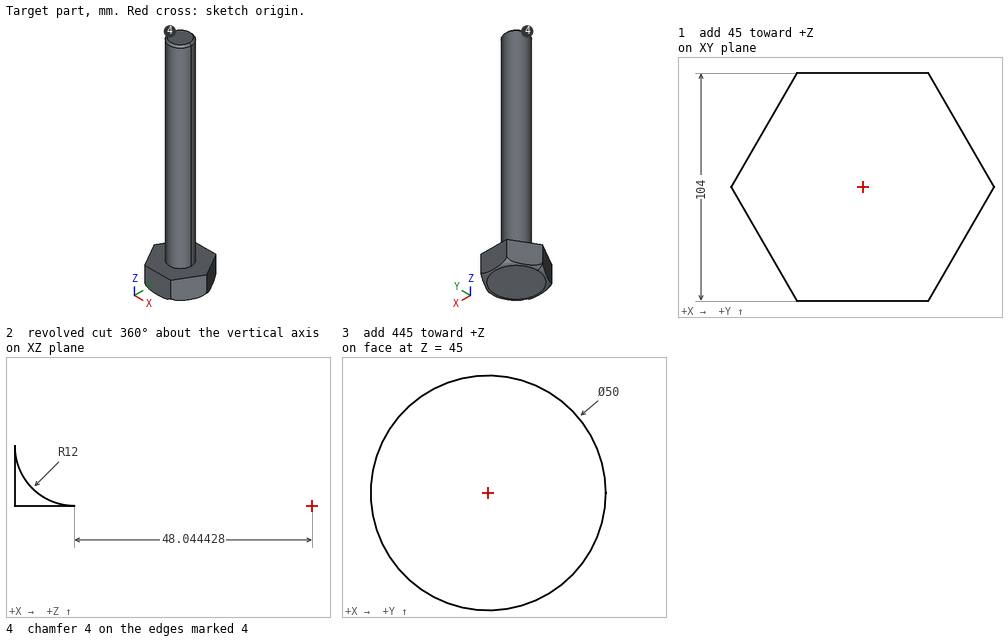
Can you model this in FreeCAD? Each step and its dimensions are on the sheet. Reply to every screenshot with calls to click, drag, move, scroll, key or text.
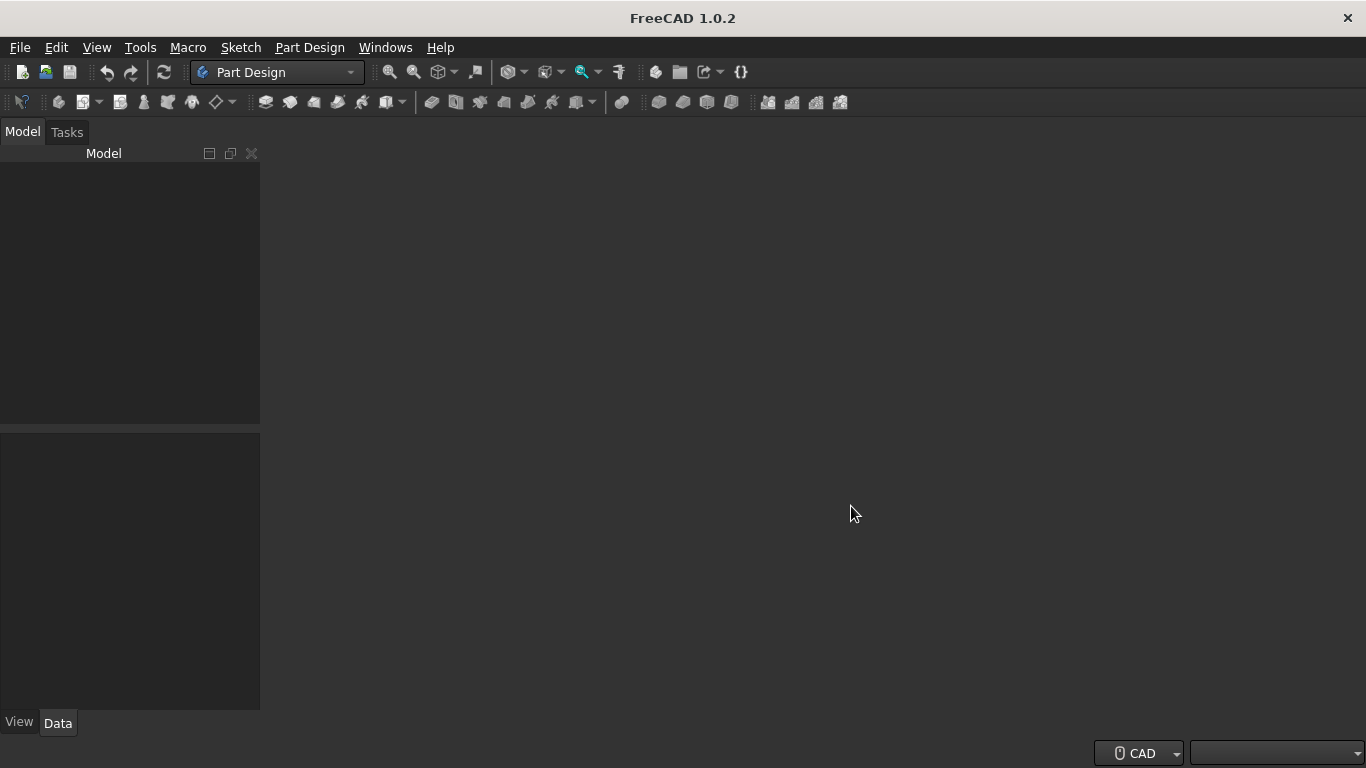
click(22, 72)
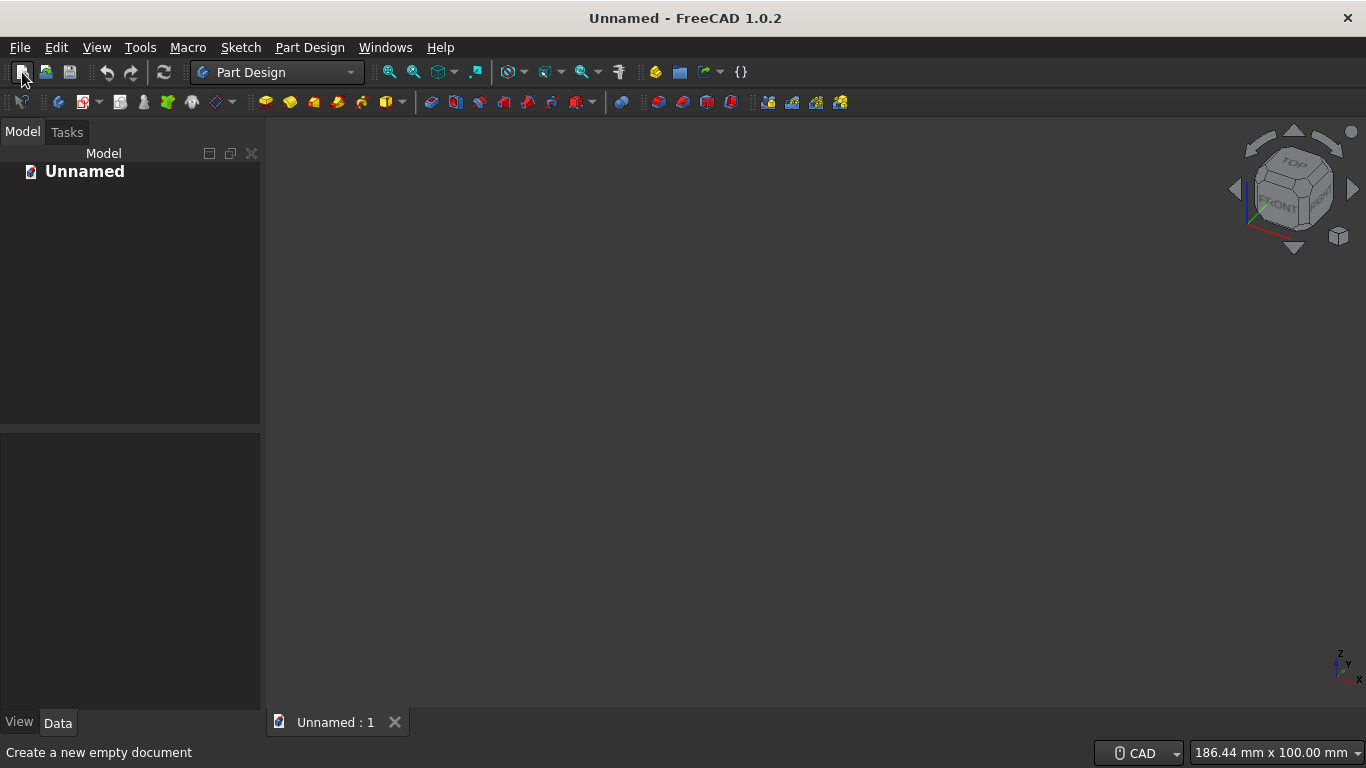
click(84, 102)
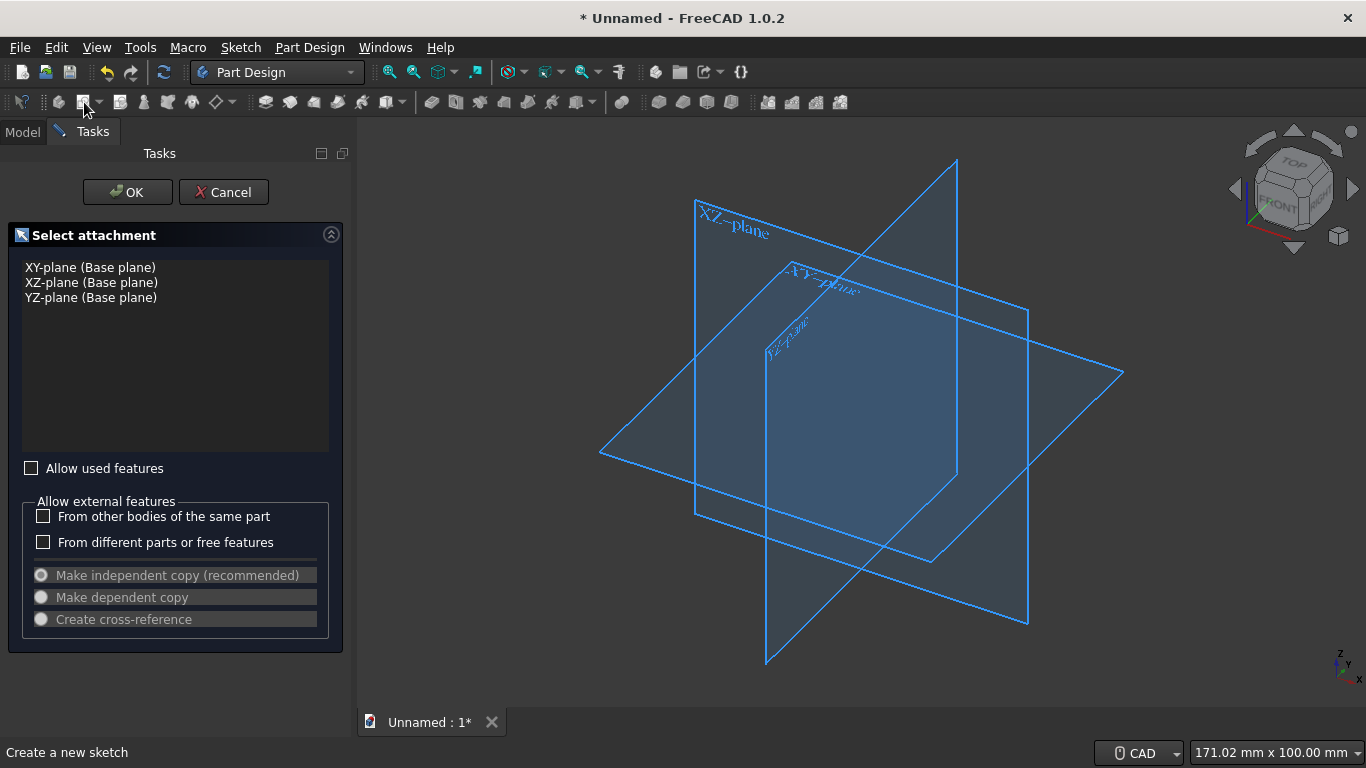
click(82, 268)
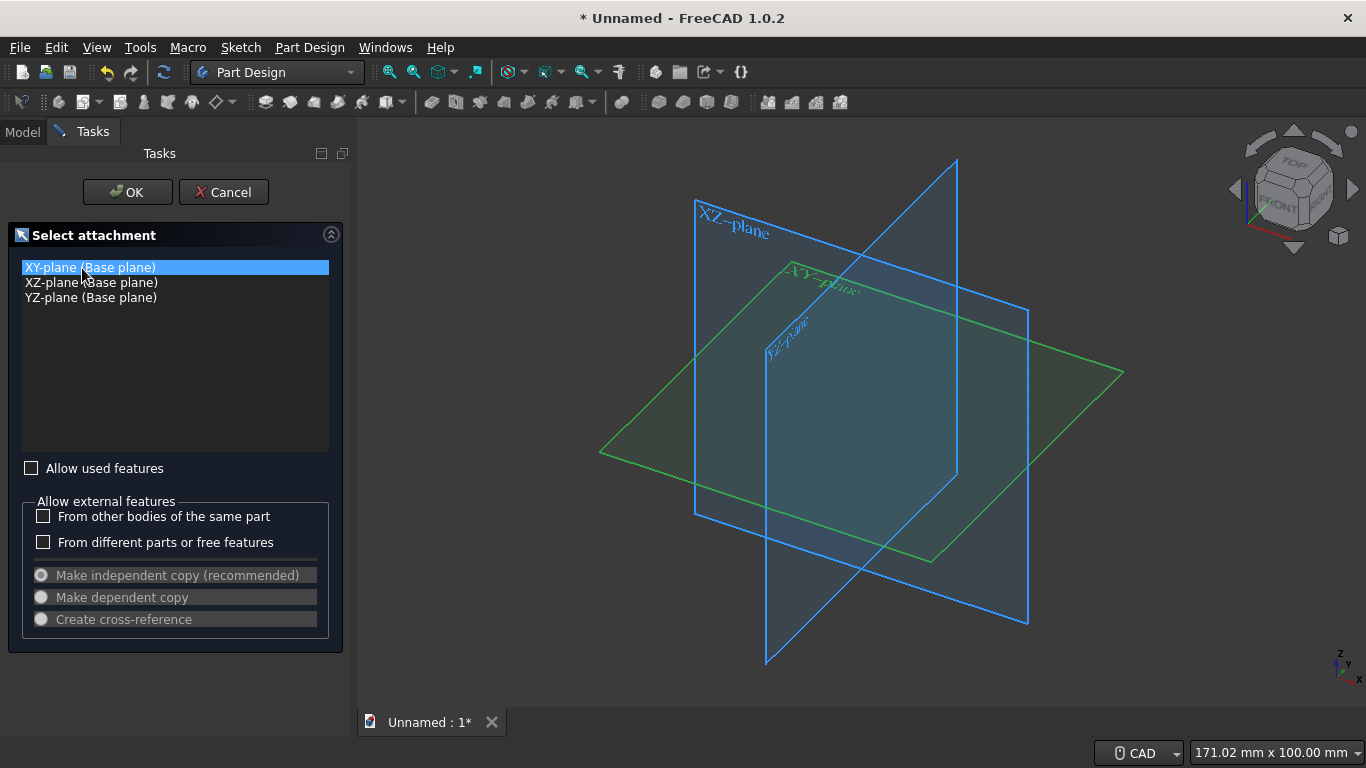
click(128, 192)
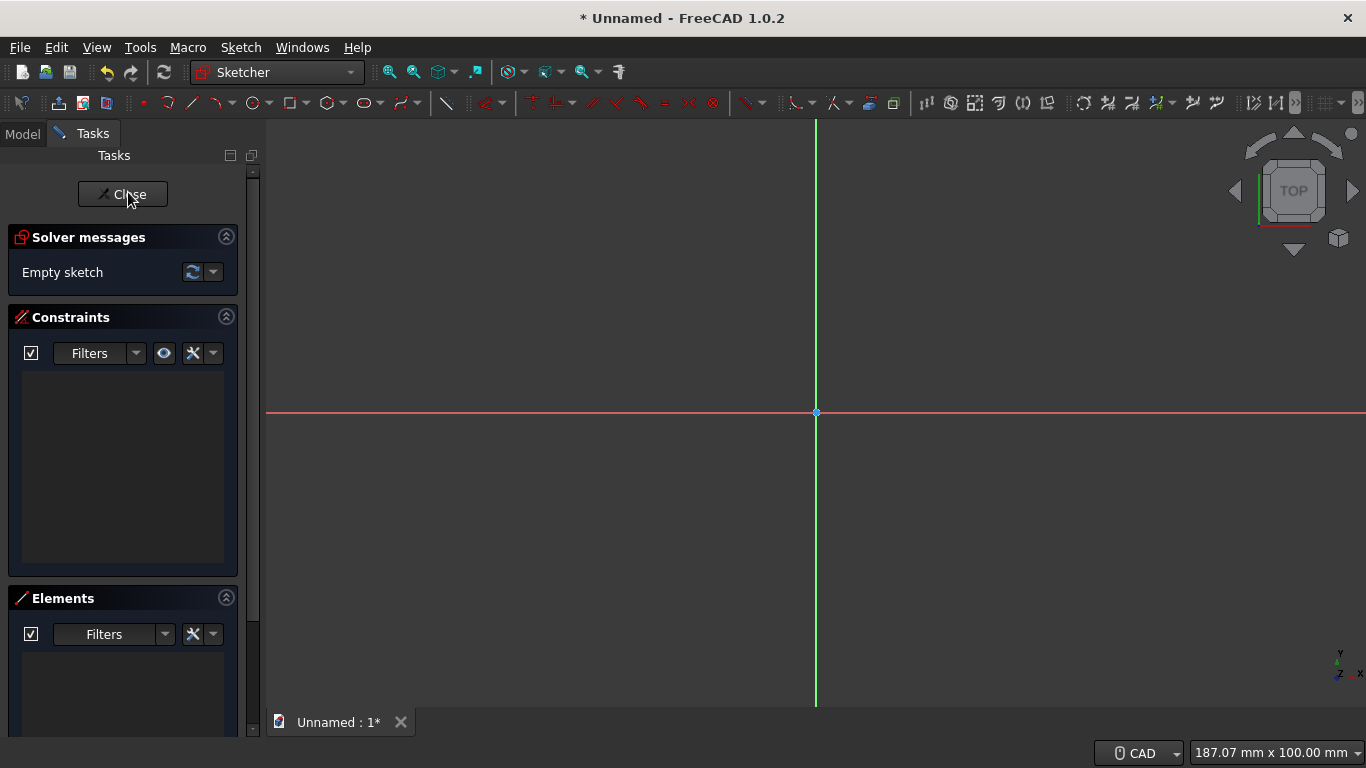
scroll(608, 413, down, 2)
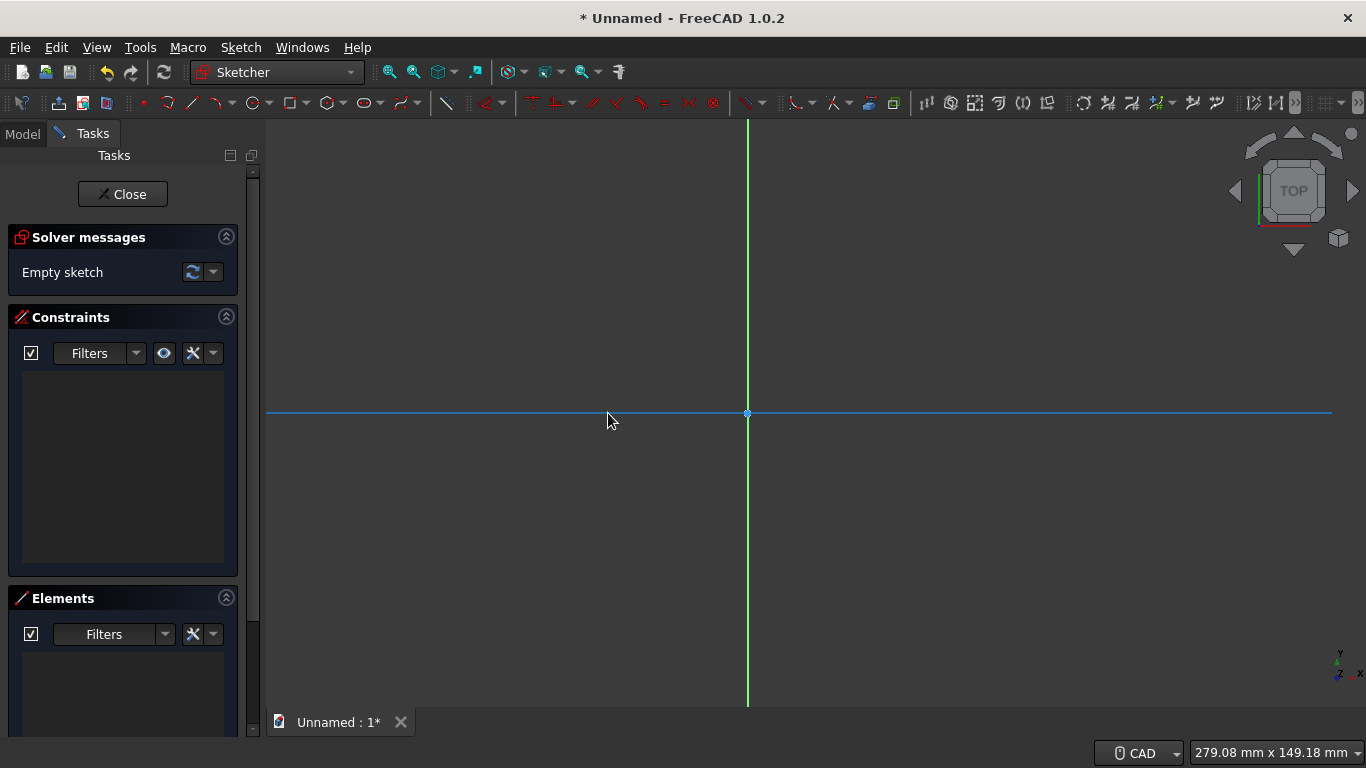
click(328, 104)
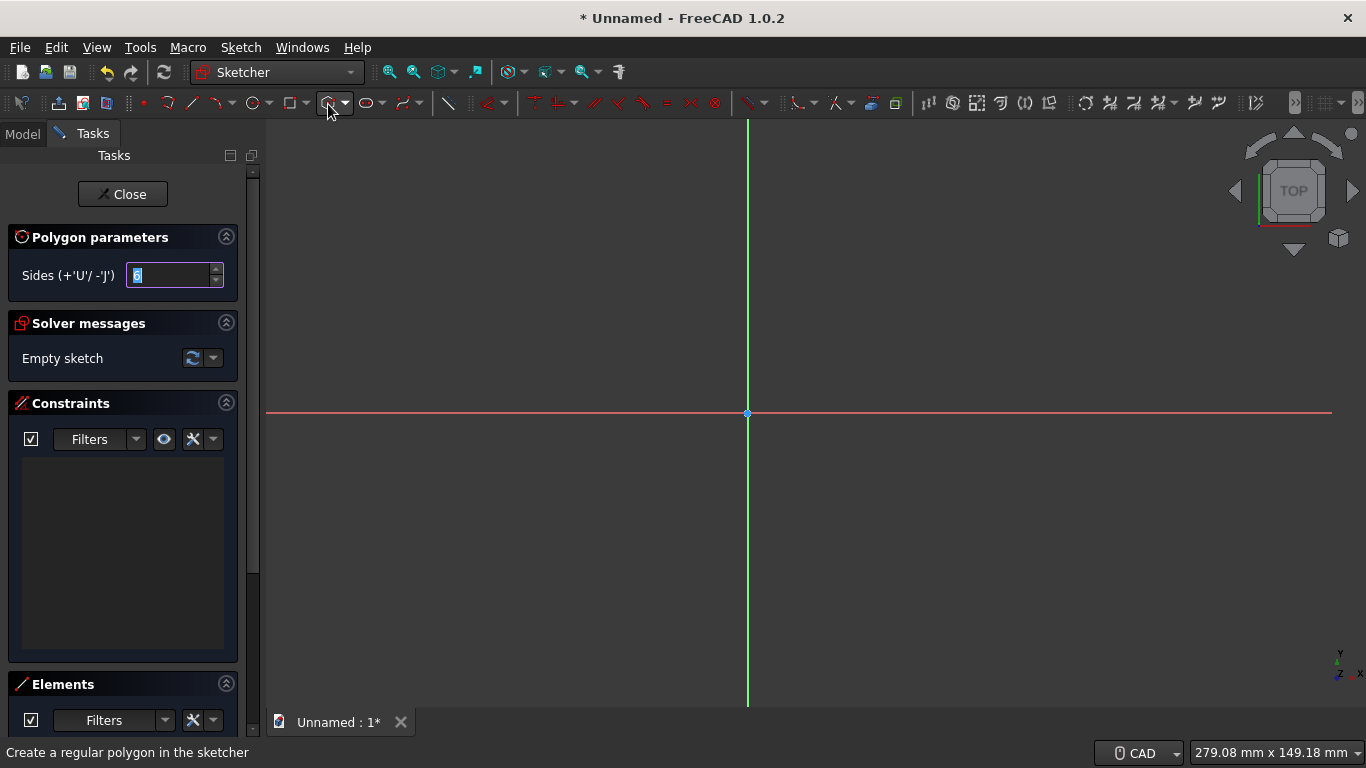
click(748, 413)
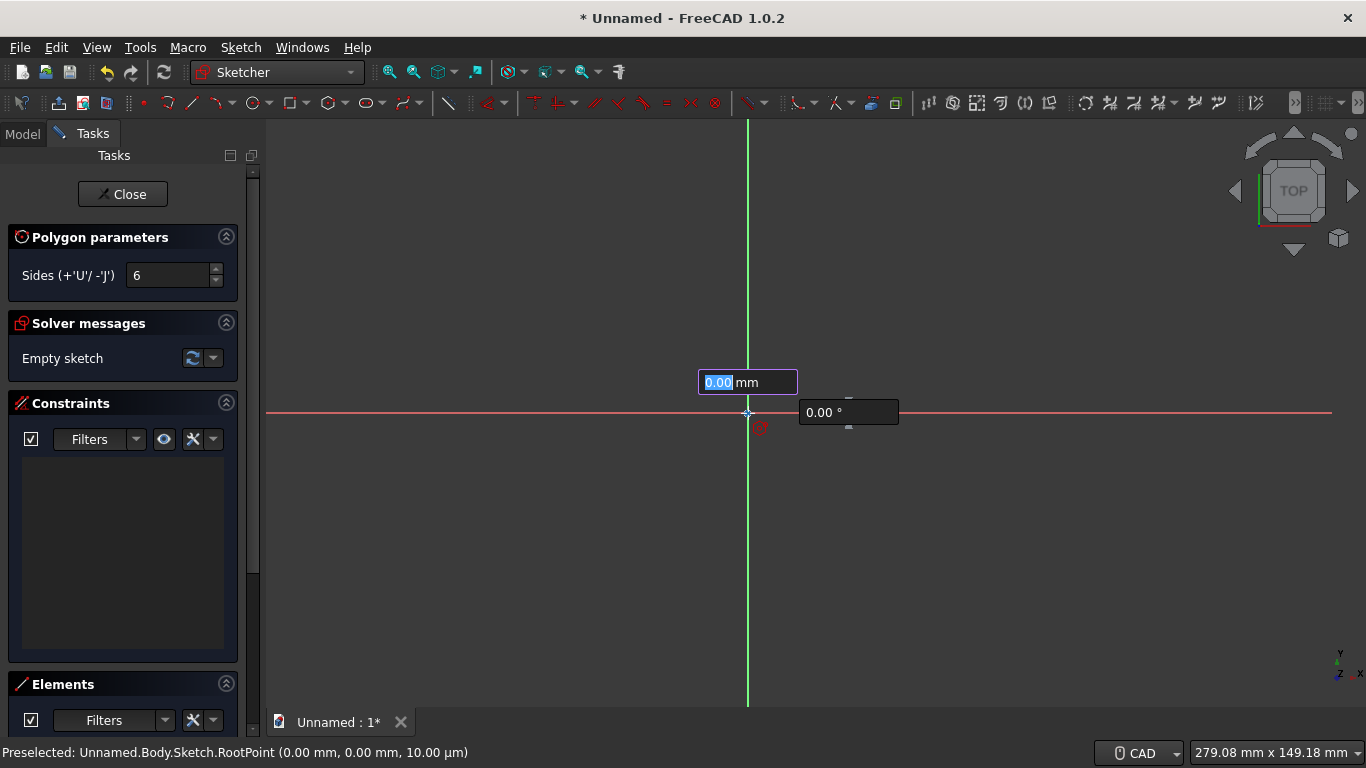
click(984, 413)
right_click(984, 413)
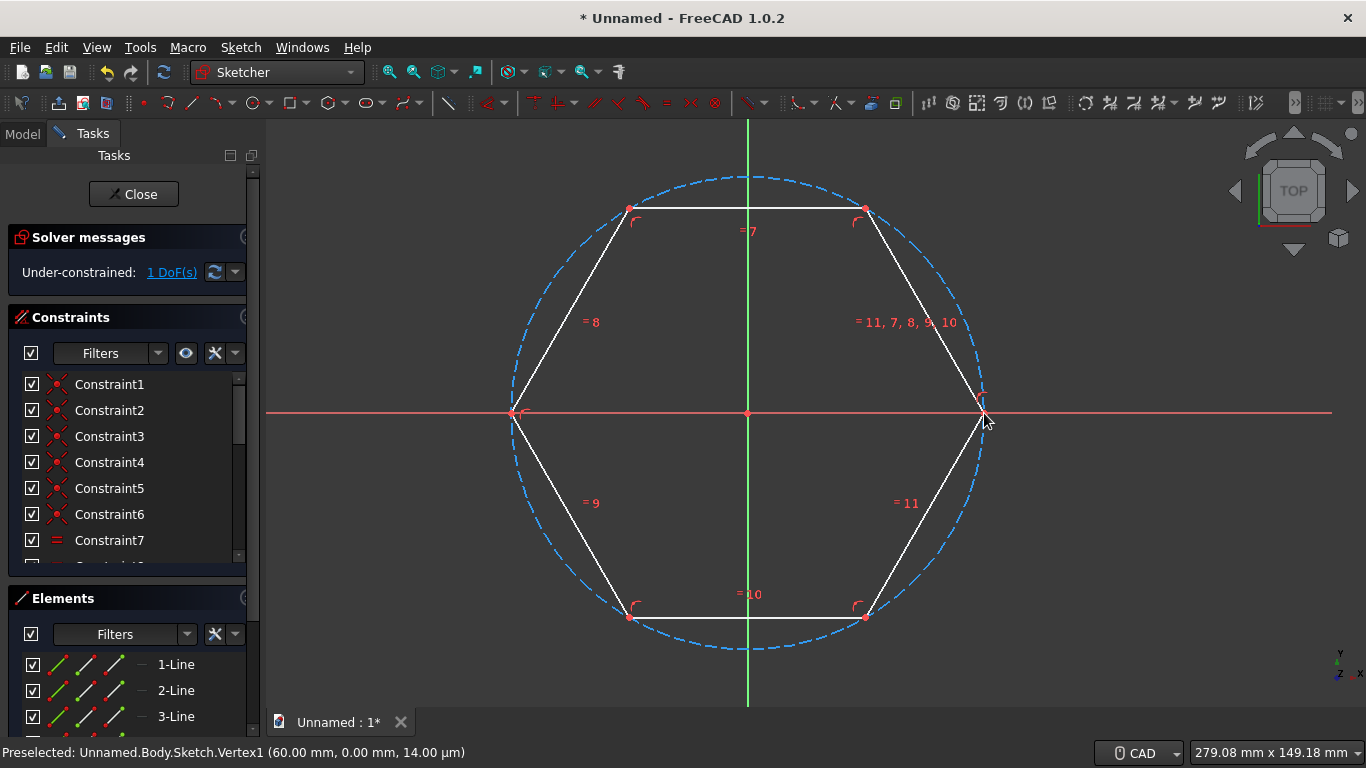
key(d)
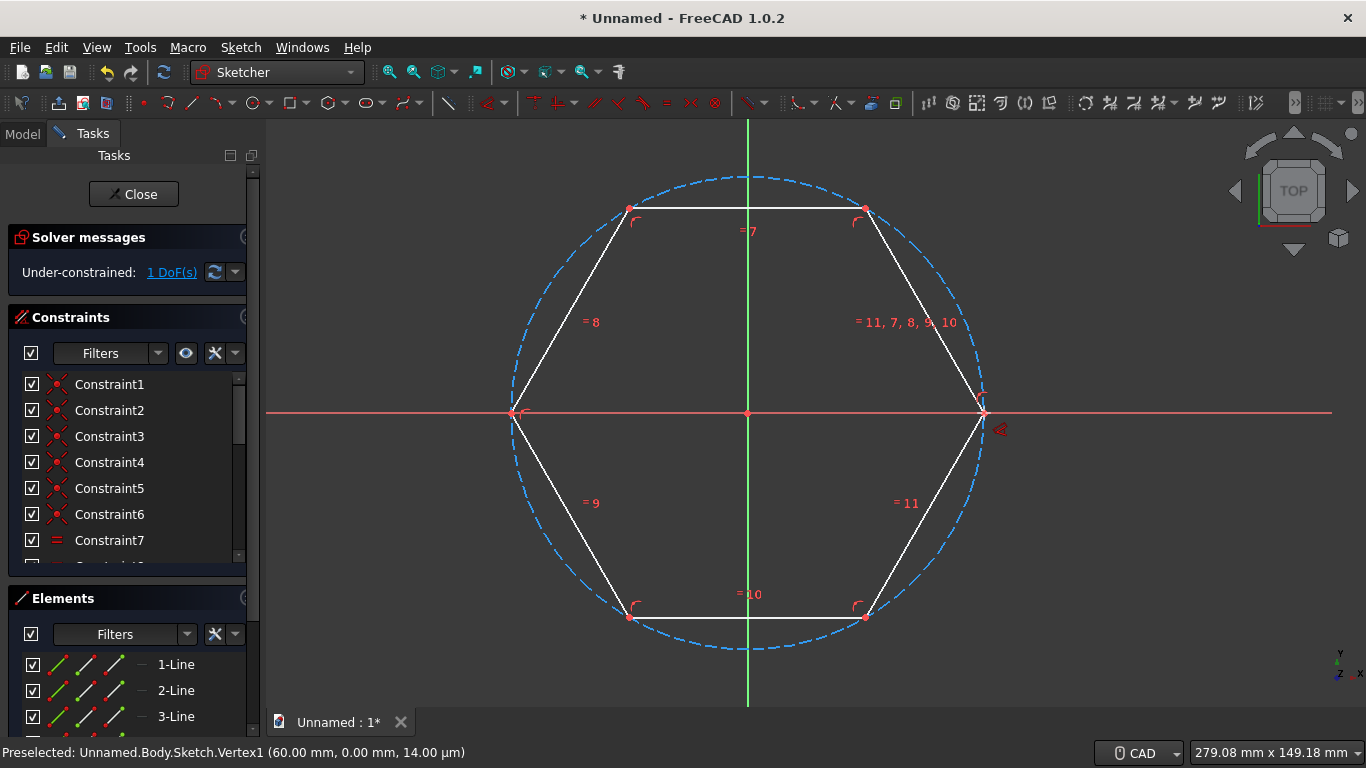
click(629, 618)